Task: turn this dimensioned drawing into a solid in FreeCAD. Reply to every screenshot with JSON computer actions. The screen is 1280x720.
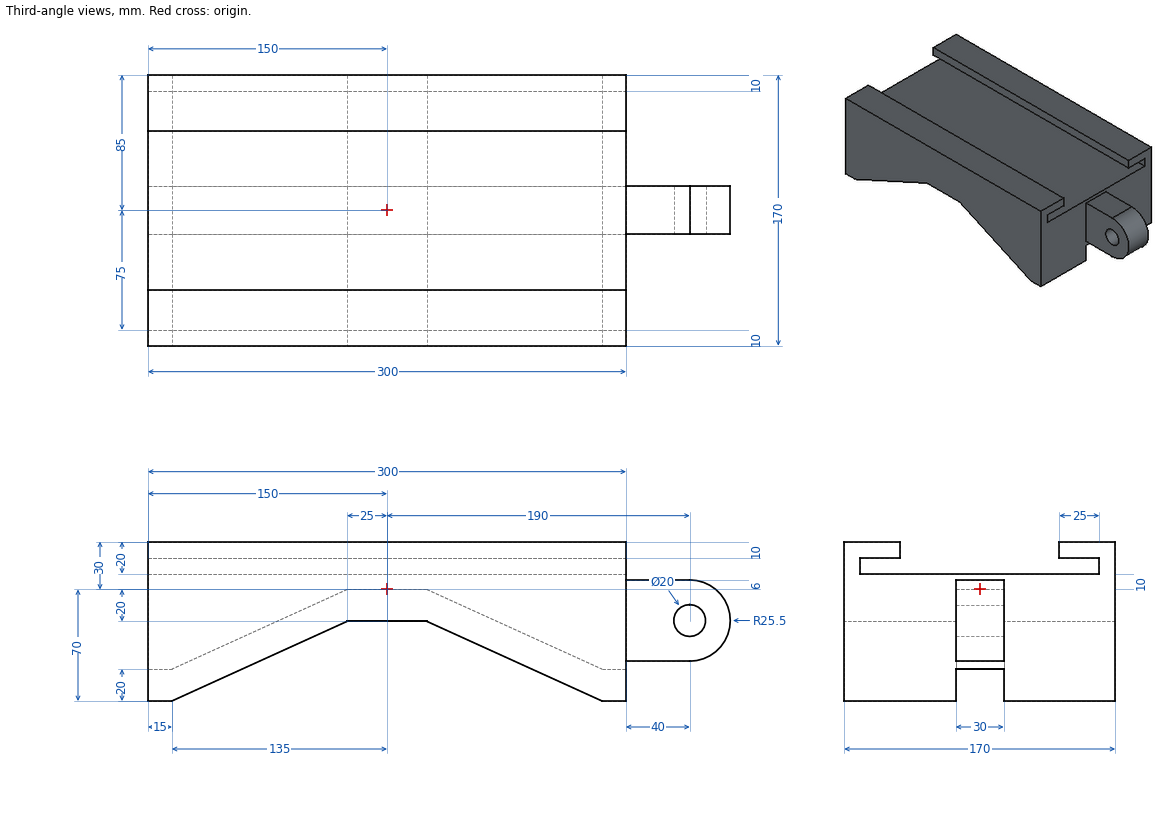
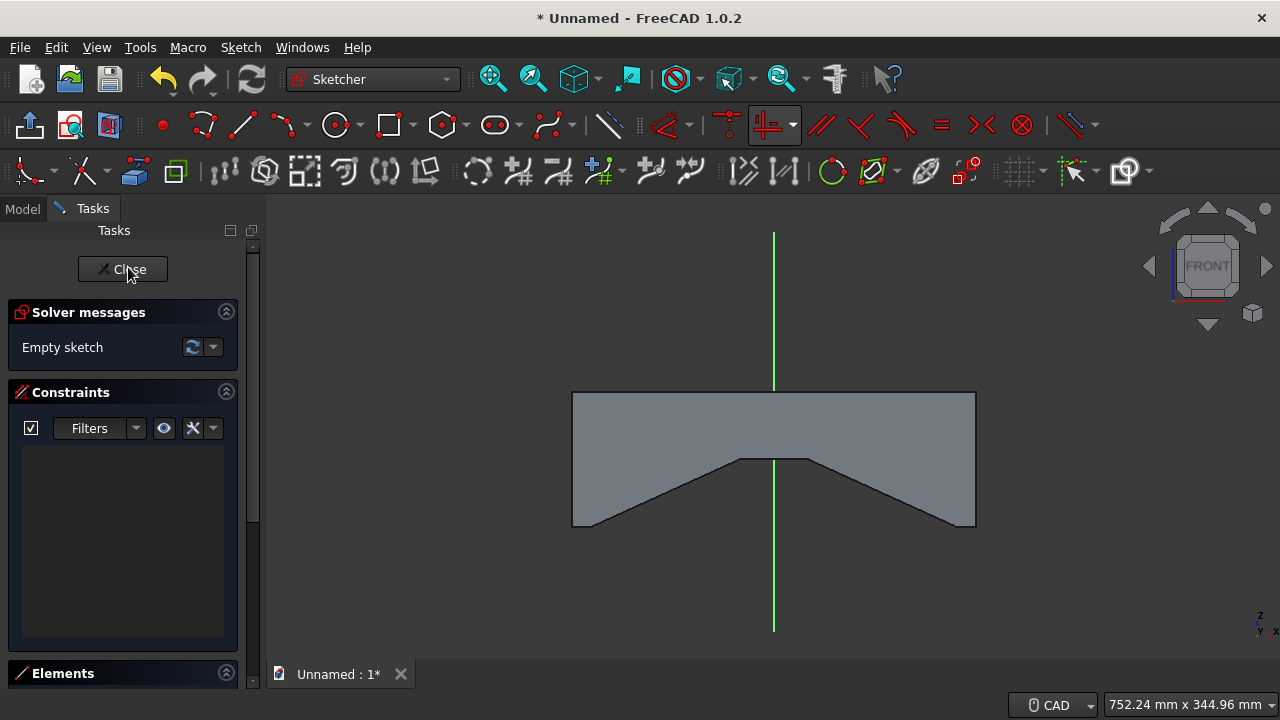
{"action": "left_click", "coordinate": [110, 126]}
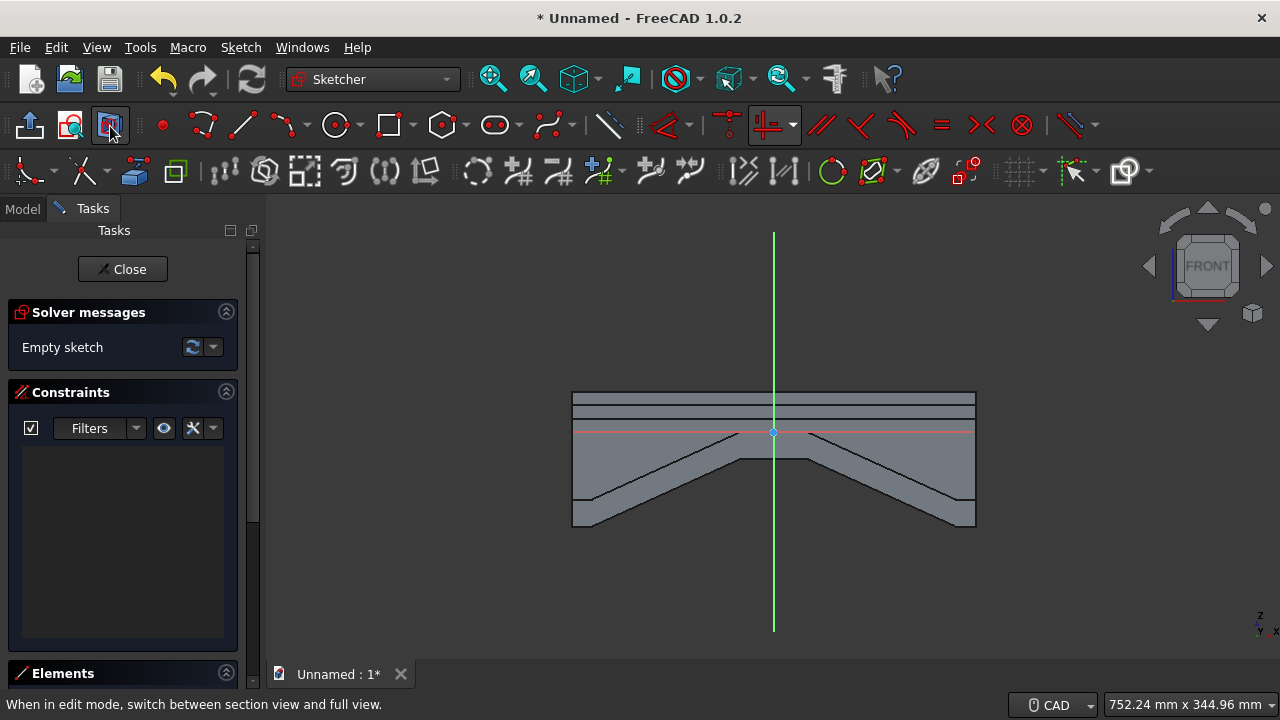
{"action": "scroll", "coordinate": [1115, 469], "scroll_direction": "up", "scroll_amount": 7}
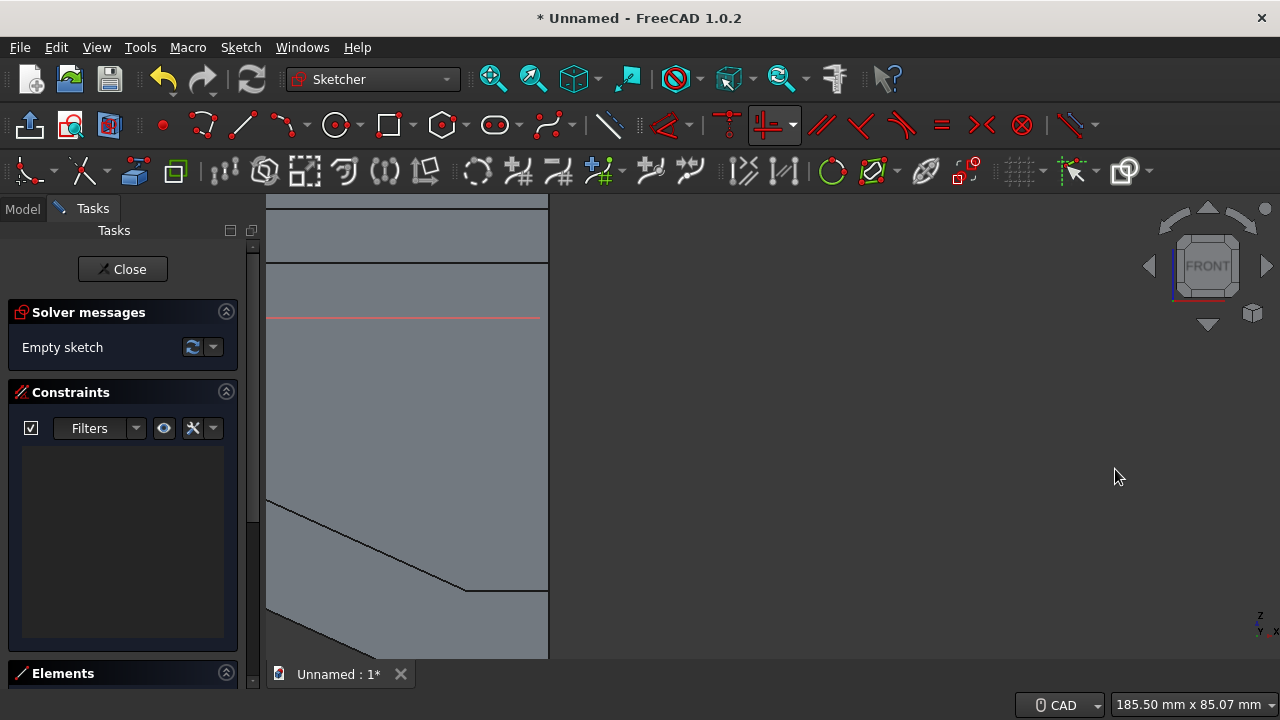
{"action": "left_click", "coordinate": [204, 126]}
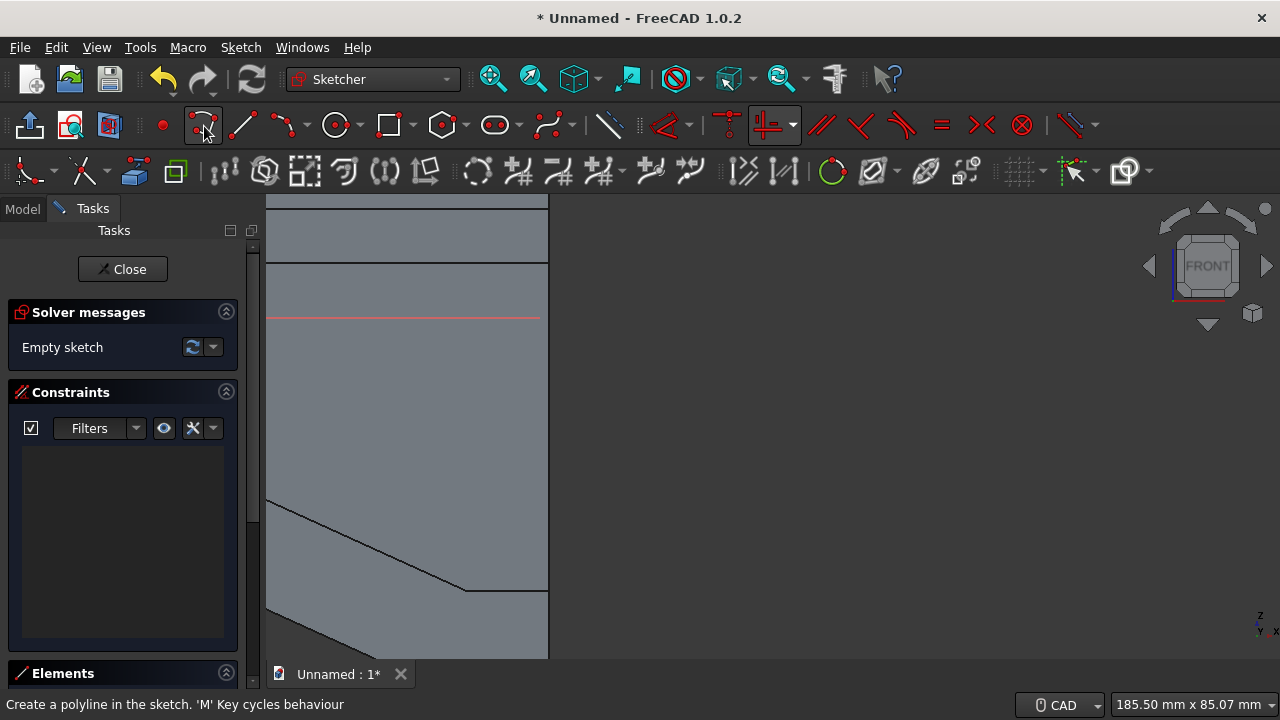
{"action": "left_click", "coordinate": [767, 564]}
{"action": "left_click", "coordinate": [549, 564]}
{"action": "left_click", "coordinate": [549, 285]}
{"action": "left_click", "coordinate": [767, 285]}
{"action": "right_click", "coordinate": [767, 285]}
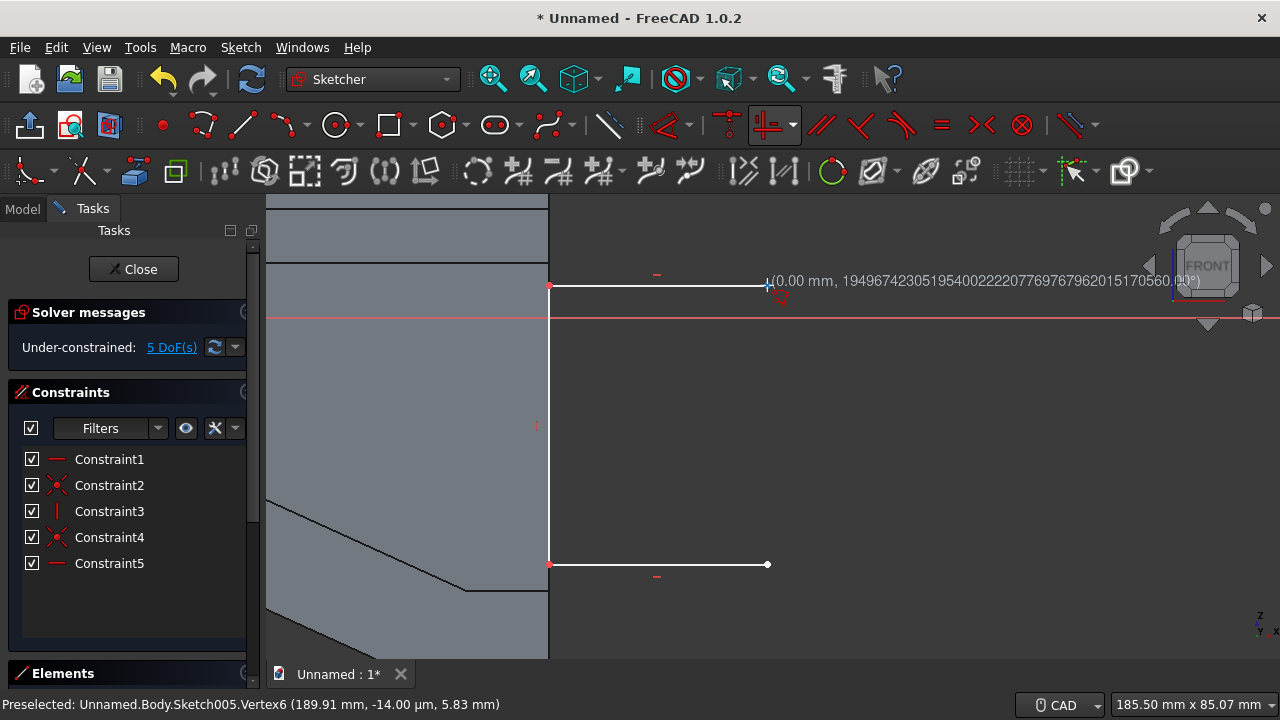
{"action": "key", "text": "g 3 a"}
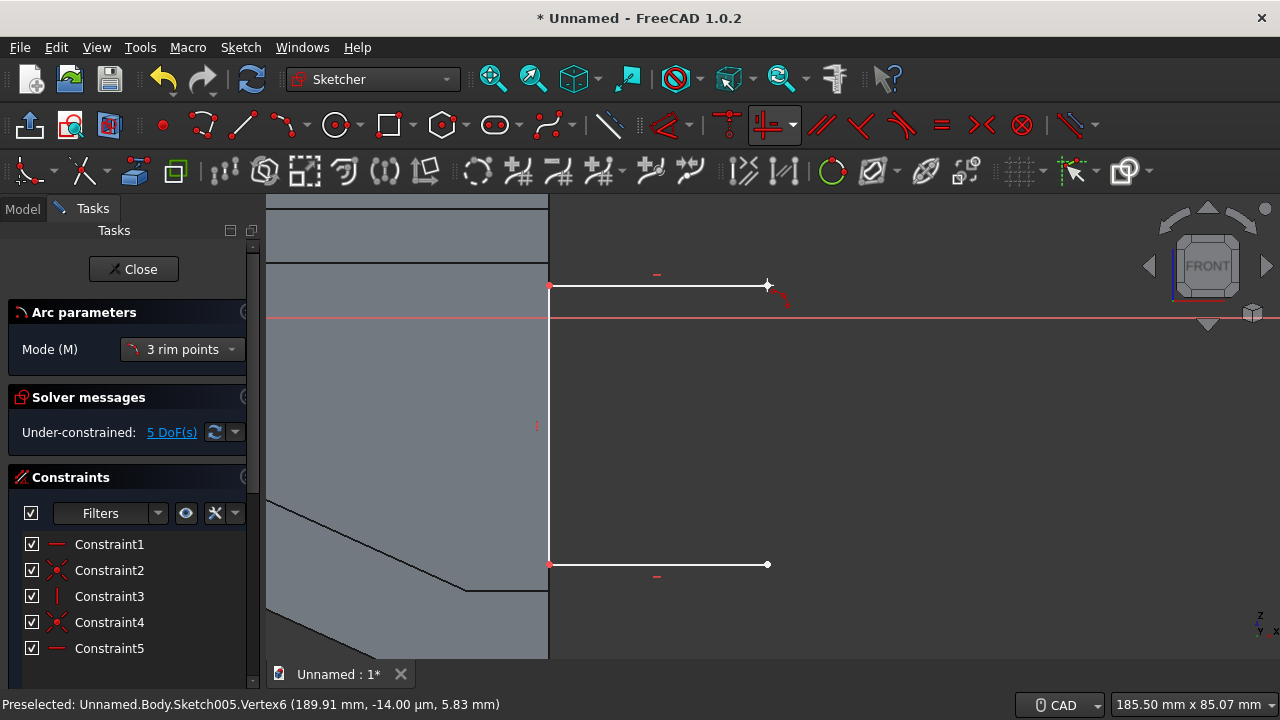
{"action": "left_click", "coordinate": [767, 286]}
{"action": "left_click", "coordinate": [767, 565]}
{"action": "left_click", "coordinate": [907, 424]}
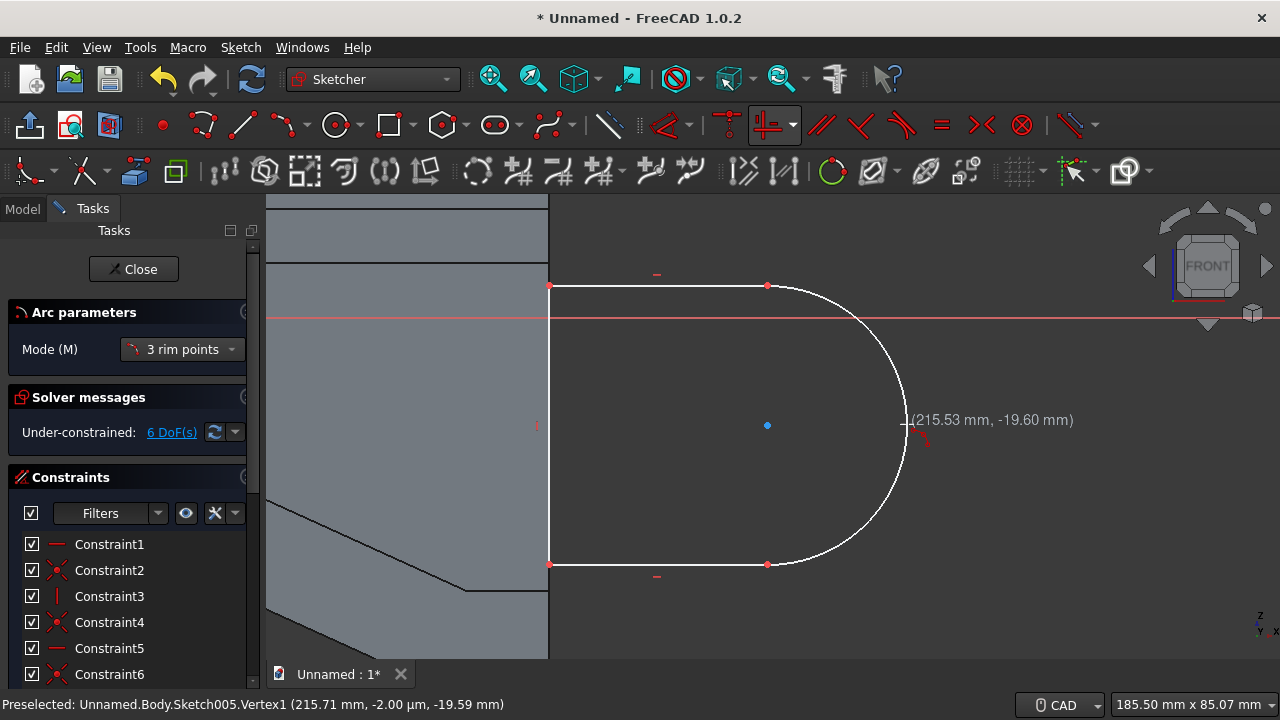
{"action": "key", "text": "g c"}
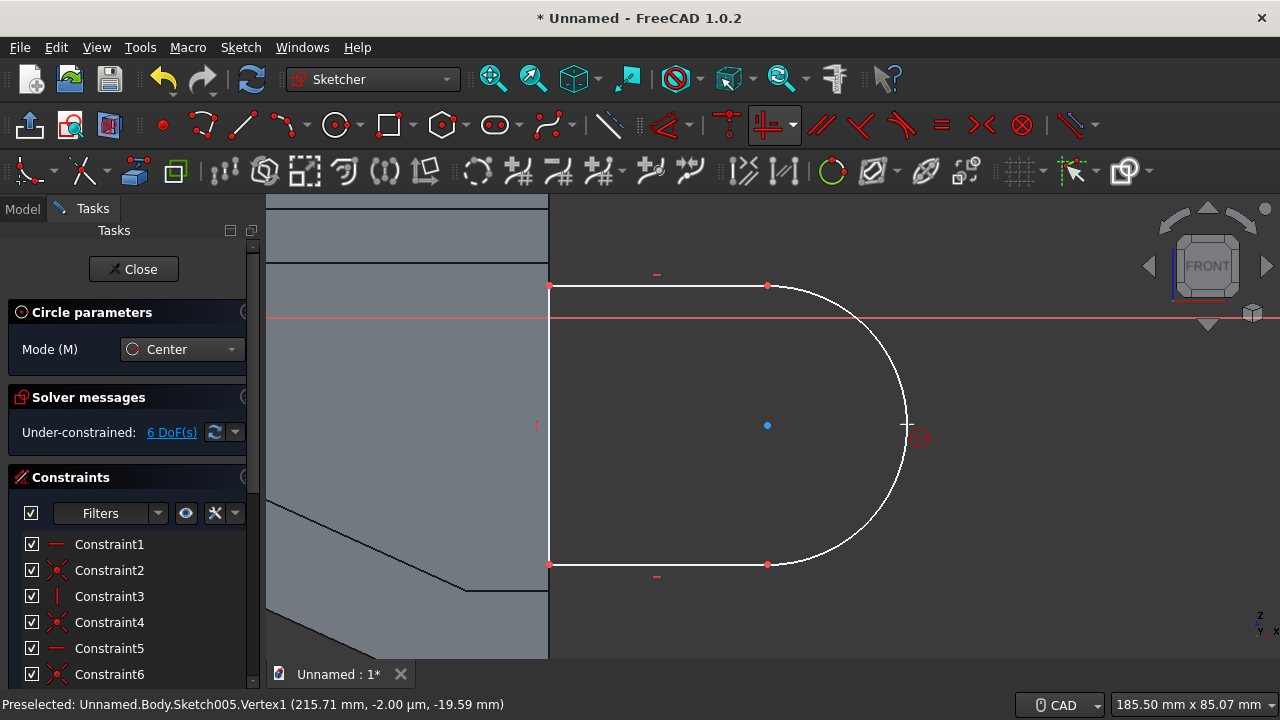
{"action": "left_click", "coordinate": [767, 424]}
{"action": "mouse_move", "coordinate": [806, 386]}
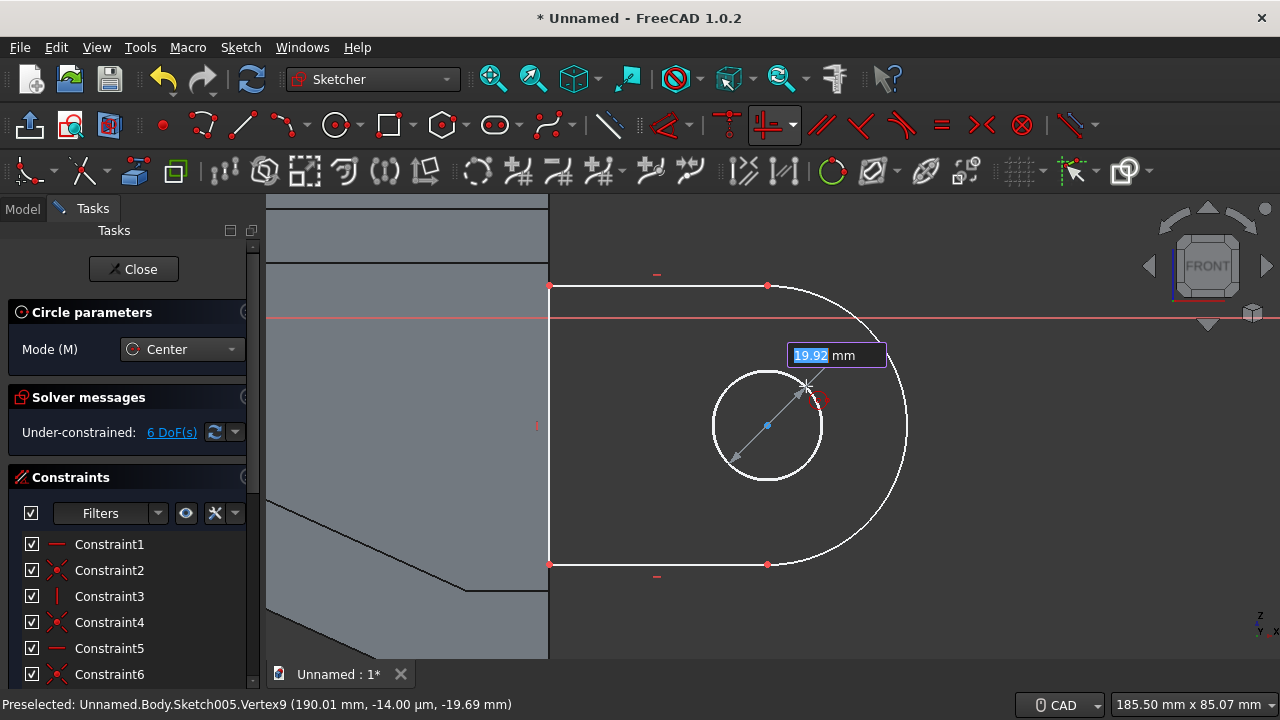
{"action": "type", "text": "20"}
{"action": "key", "text": "Return"}
{"action": "key", "text": "Escape"}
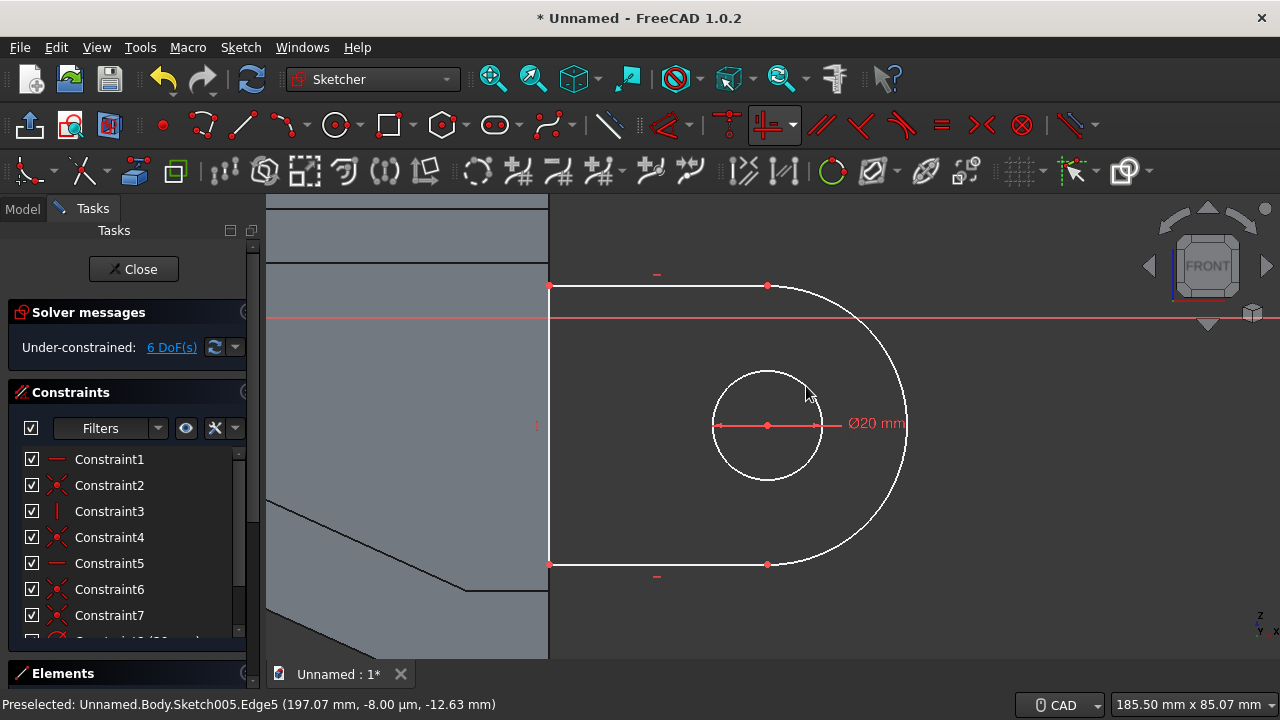
{"action": "left_click", "coordinate": [702, 565]}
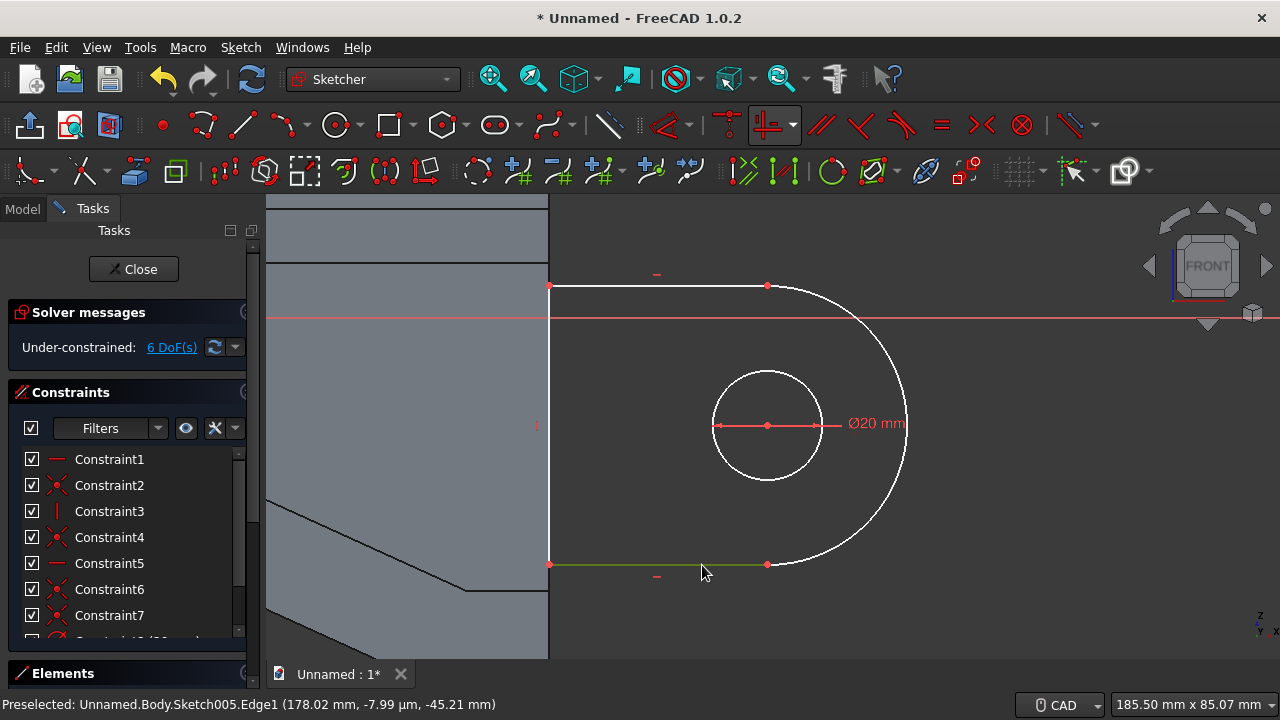
{"action": "left_click", "coordinate": [880, 508]}